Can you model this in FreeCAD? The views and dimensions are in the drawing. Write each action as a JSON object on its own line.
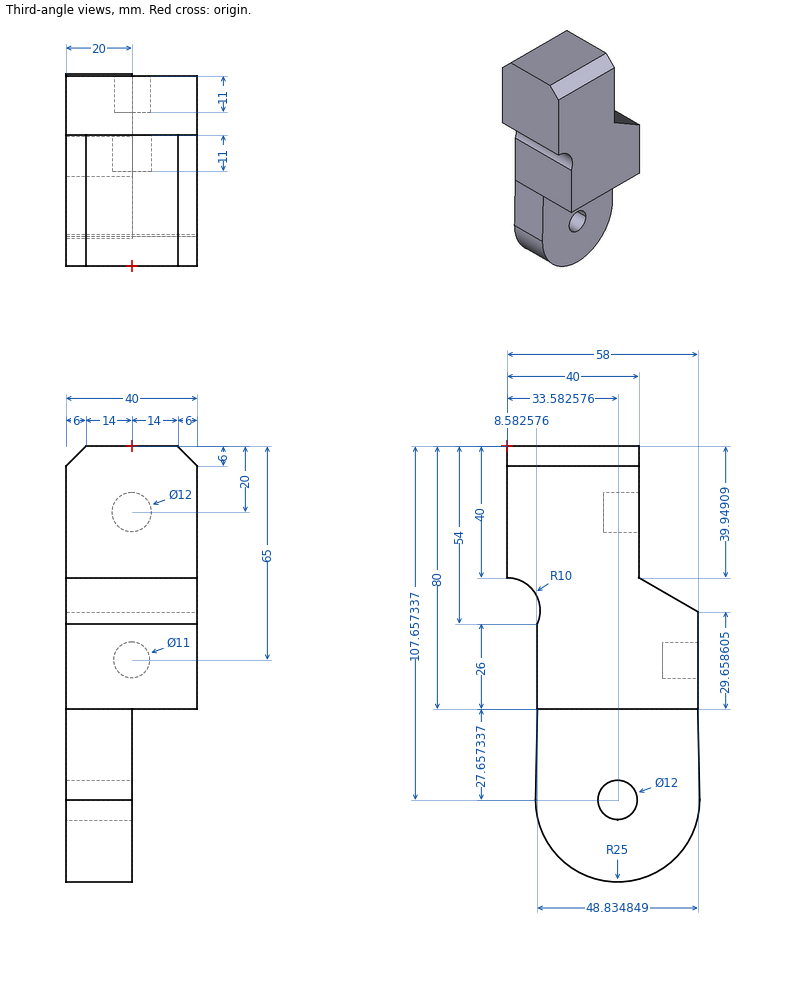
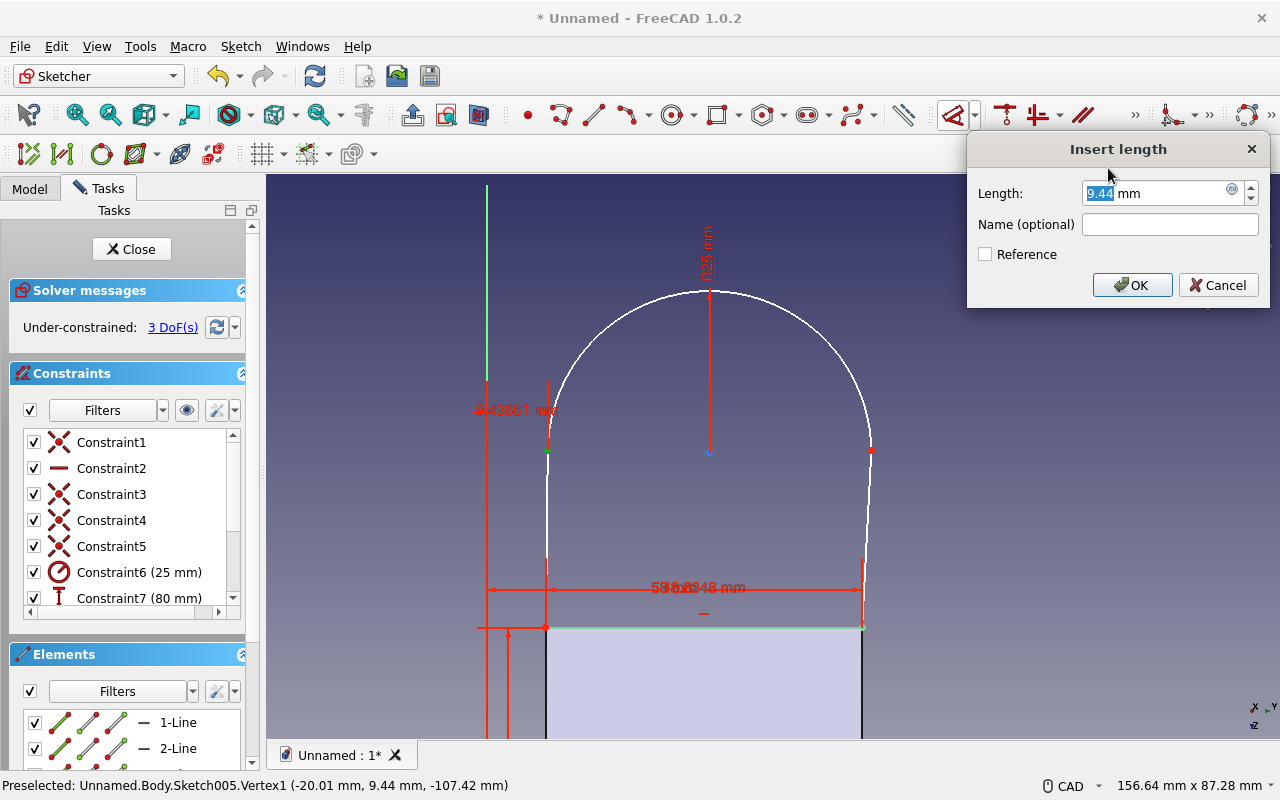
{"action": "type", "text": "8.582576"}
{"action": "key", "text": "Return"}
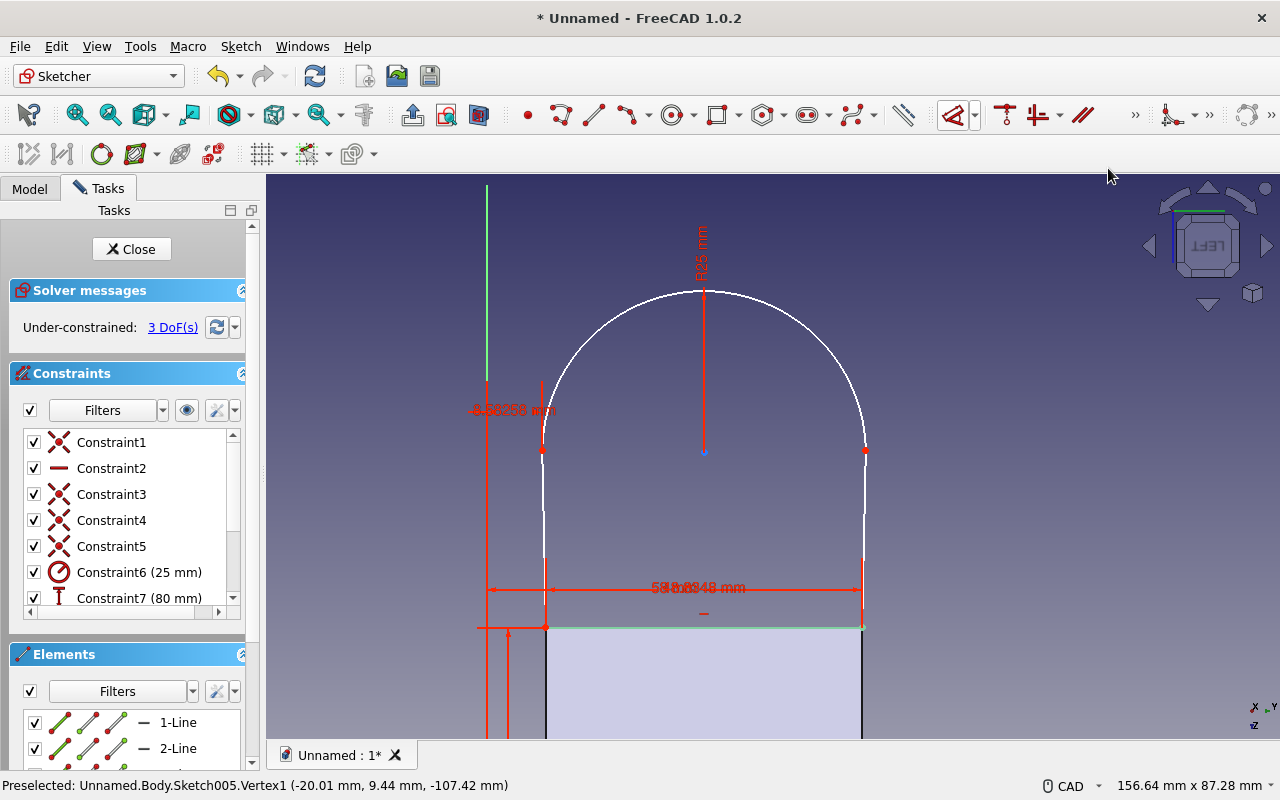
{"action": "left_click", "coordinate": [543, 503]}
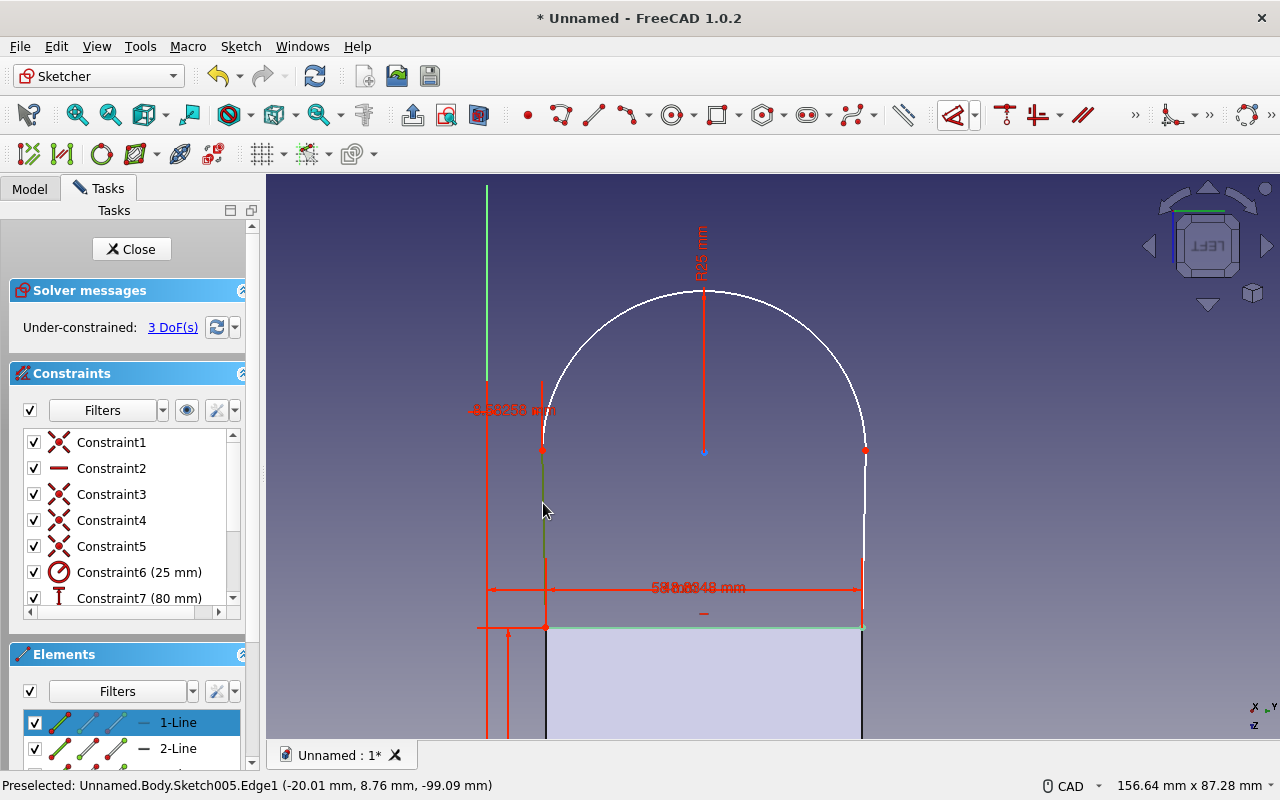
{"action": "key", "text": "i"}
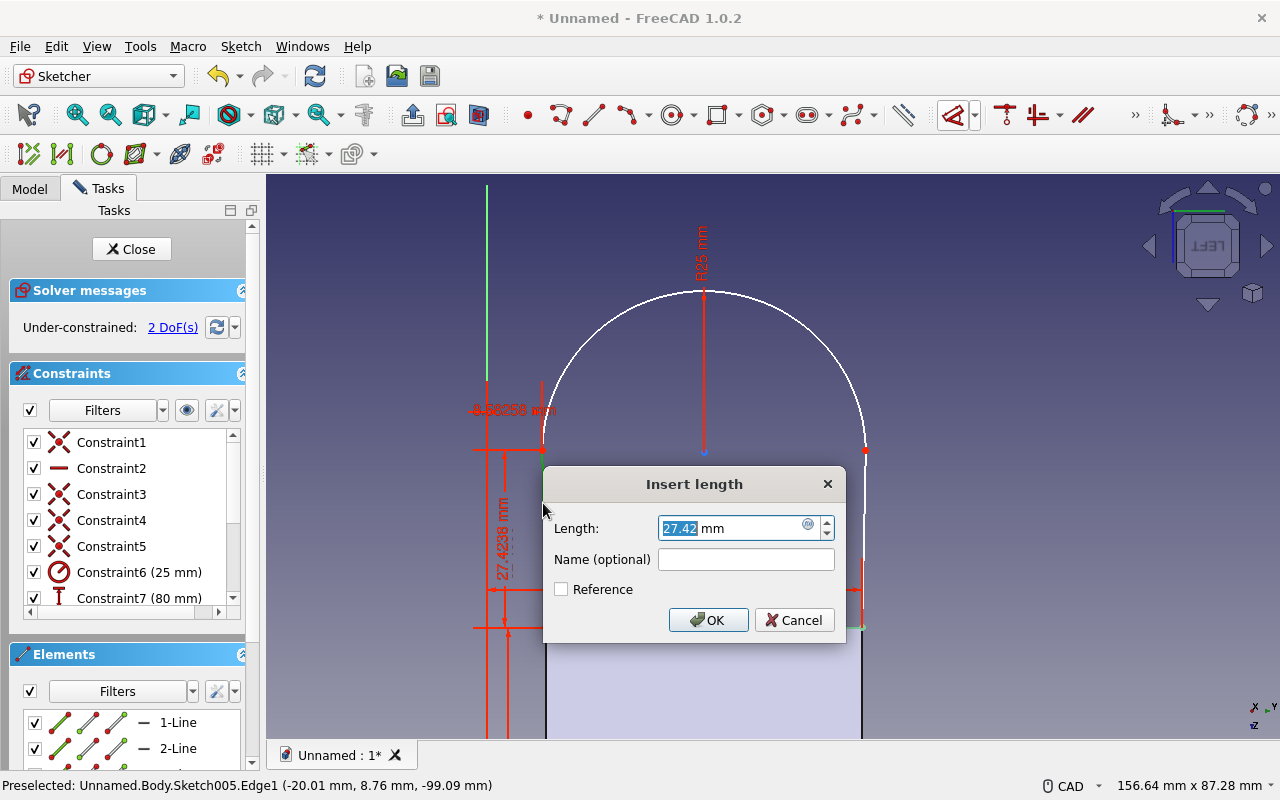
{"action": "type", "text": "27.657337"}
{"action": "key", "text": "Return"}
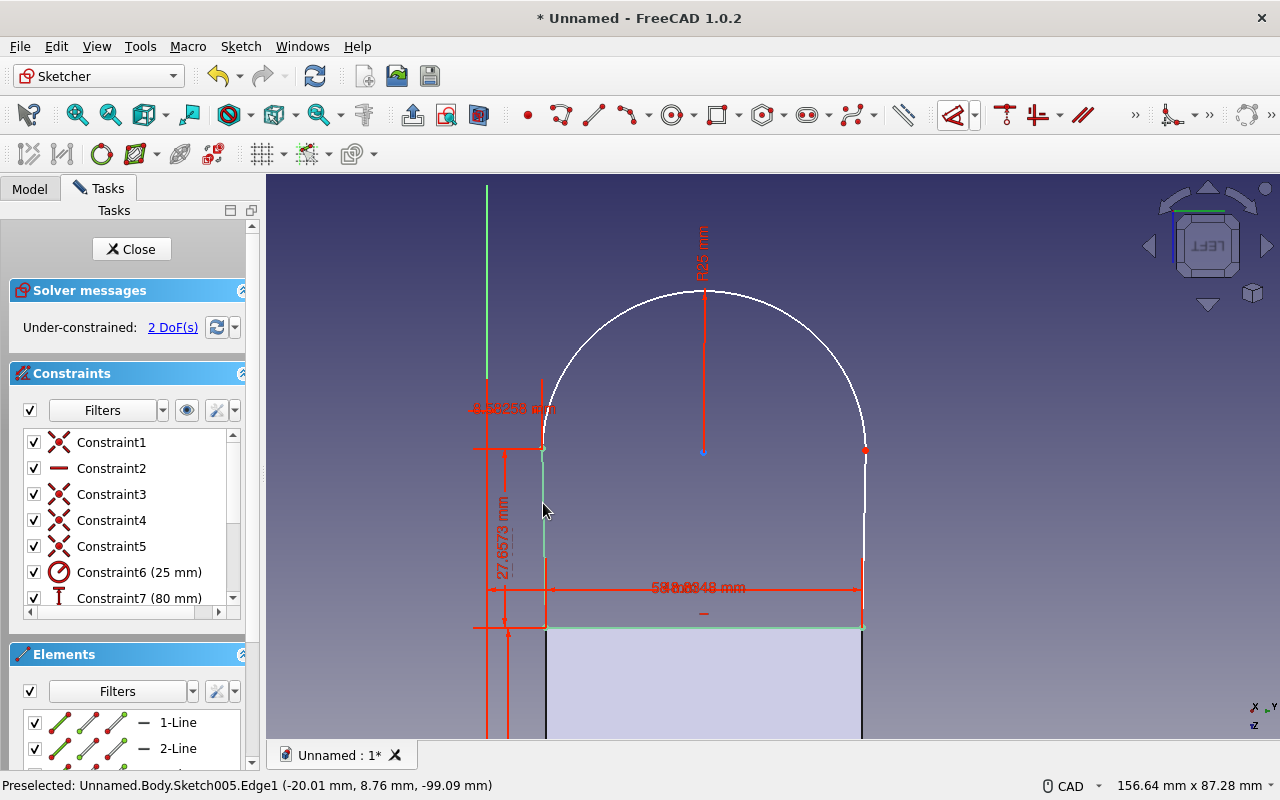
{"action": "left_click", "coordinate": [863, 574]}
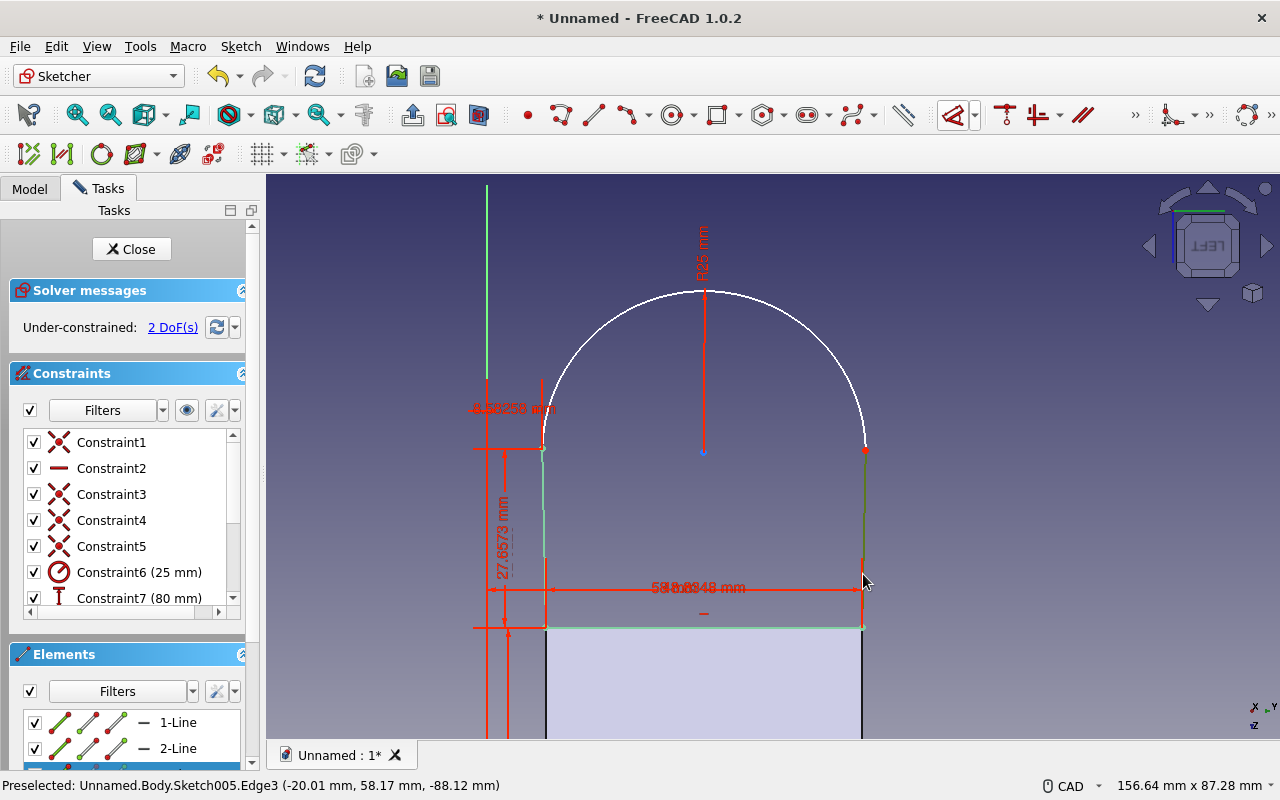
{"action": "key", "text": "i"}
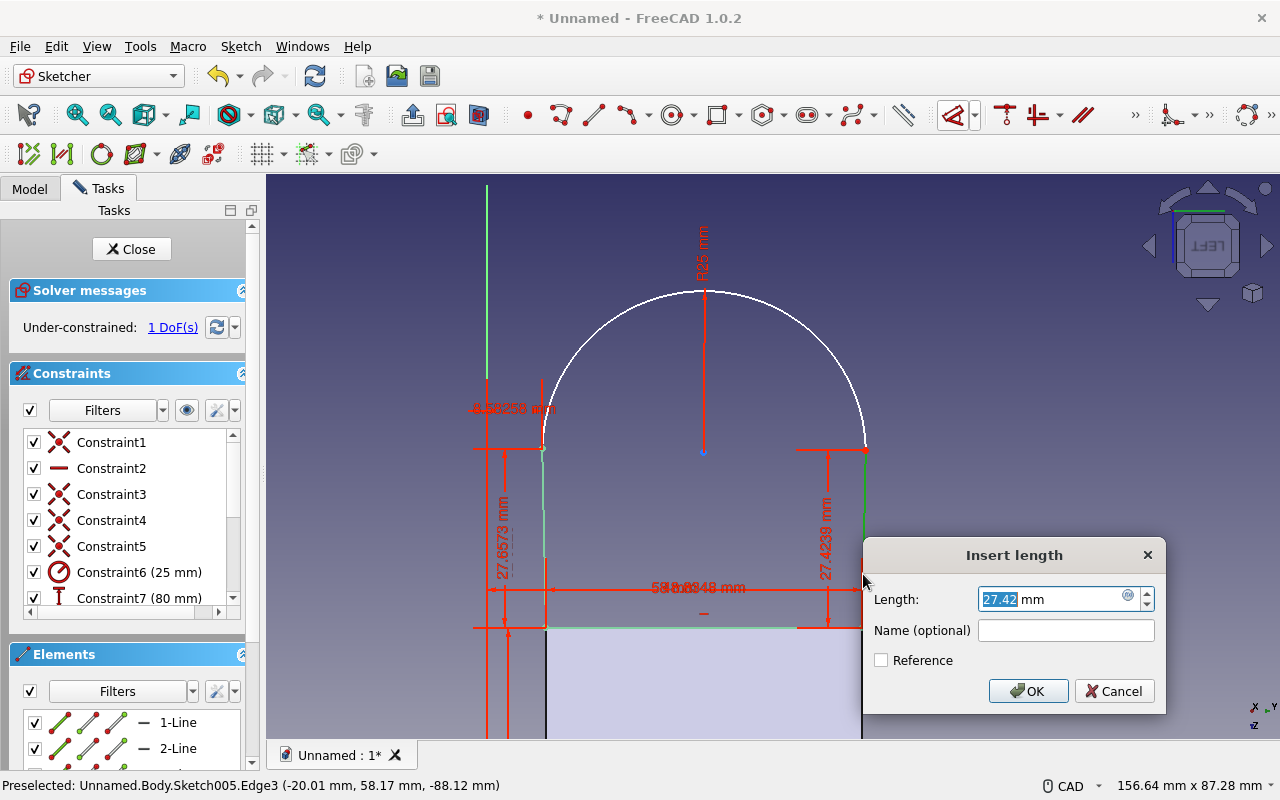
{"action": "type", "text": "27.657337"}
{"action": "key", "text": "Return"}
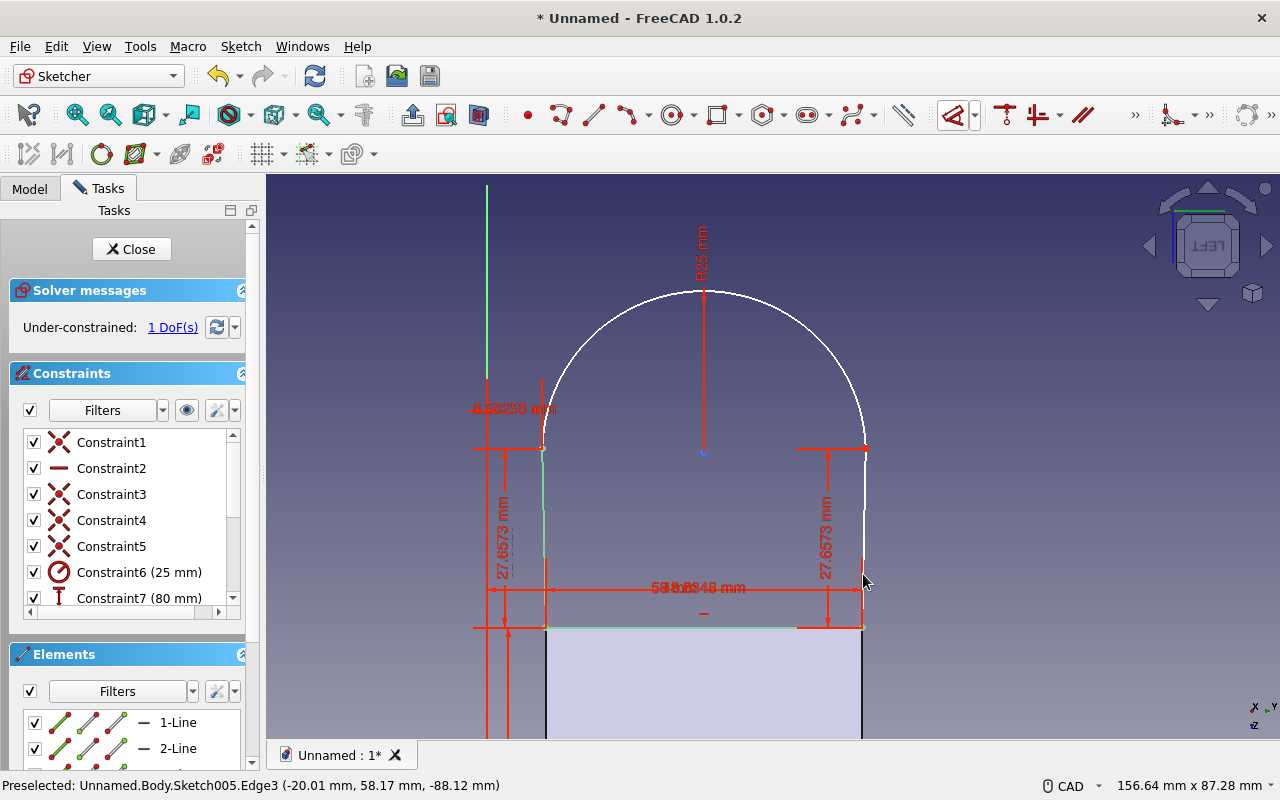
{"action": "left_click", "coordinate": [704, 453]}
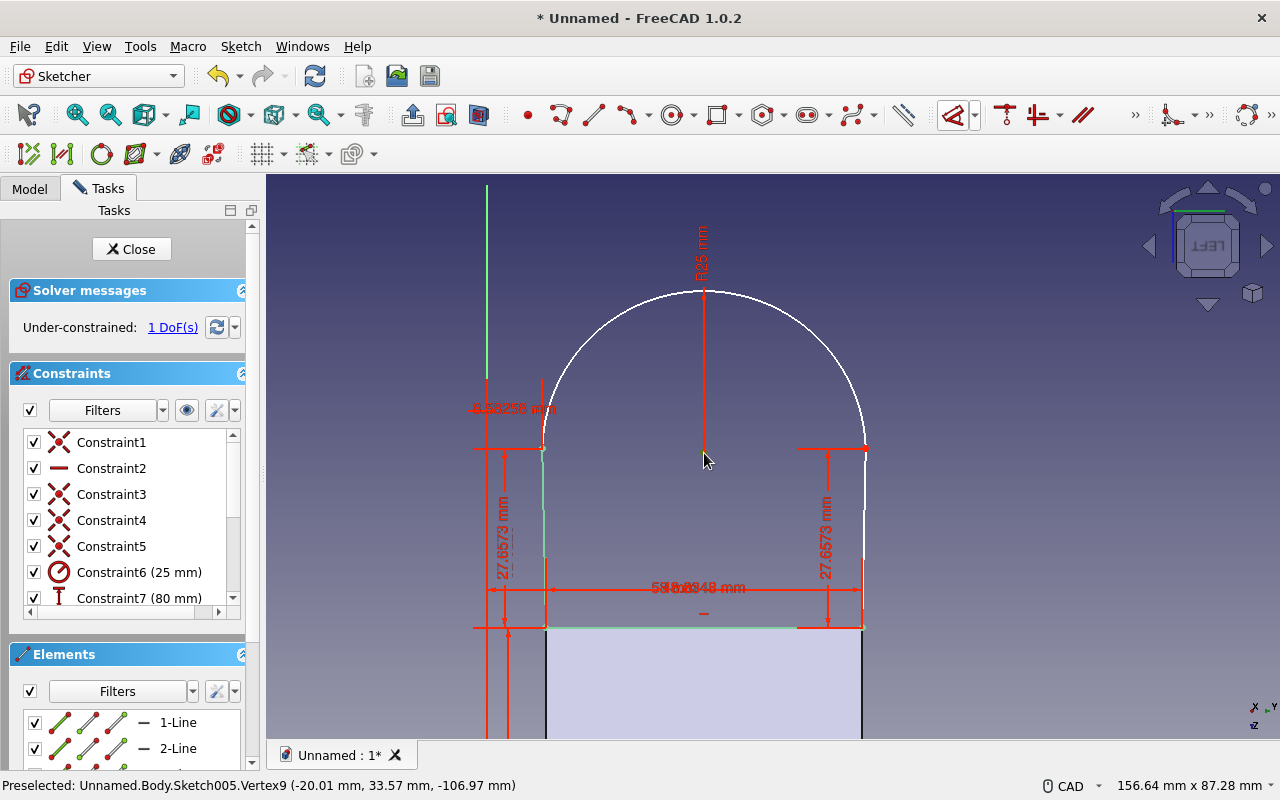
{"action": "key", "text": "i"}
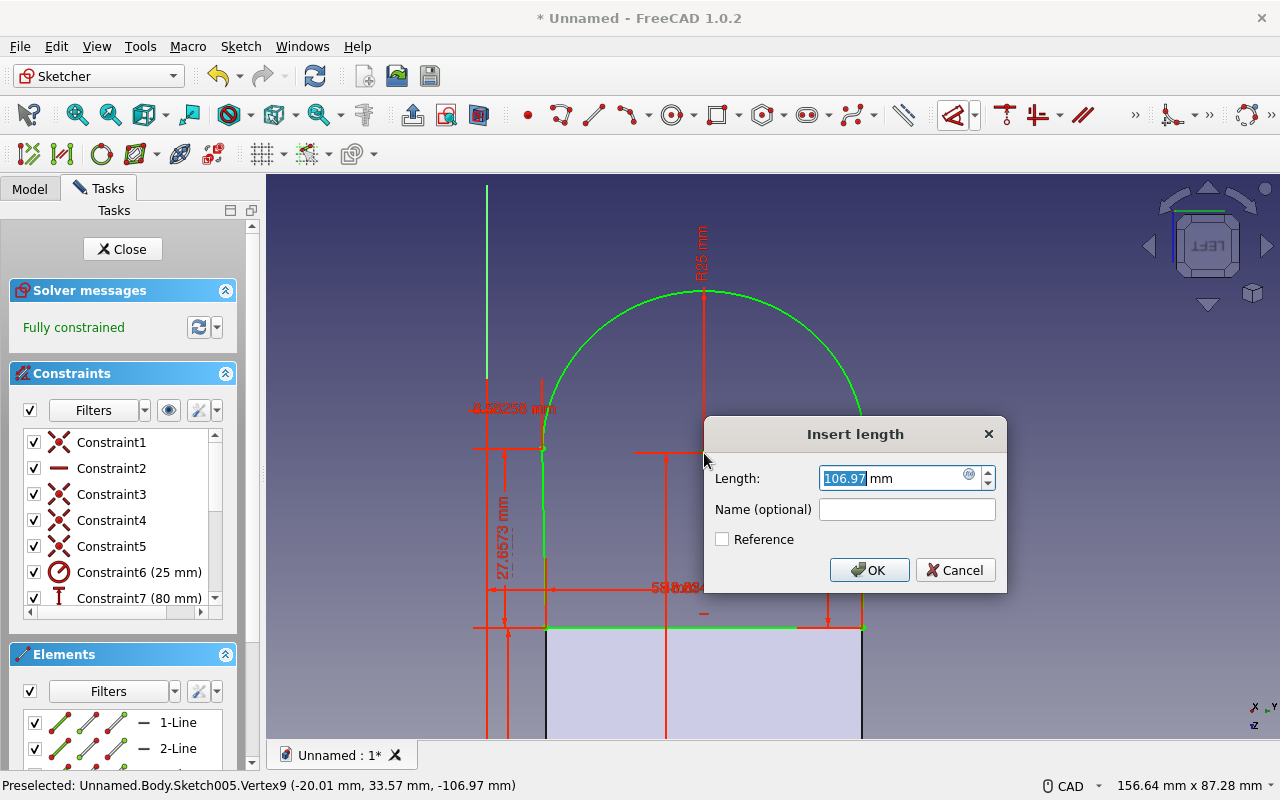
{"action": "type", "text": "107.657337"}
{"action": "key", "text": "Return"}